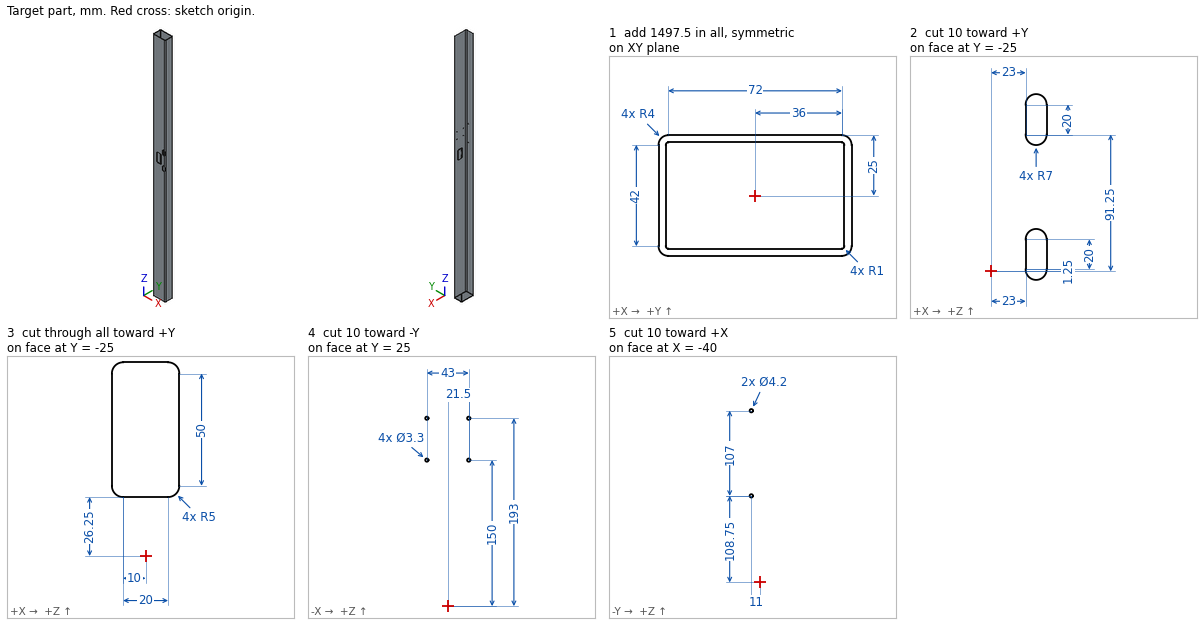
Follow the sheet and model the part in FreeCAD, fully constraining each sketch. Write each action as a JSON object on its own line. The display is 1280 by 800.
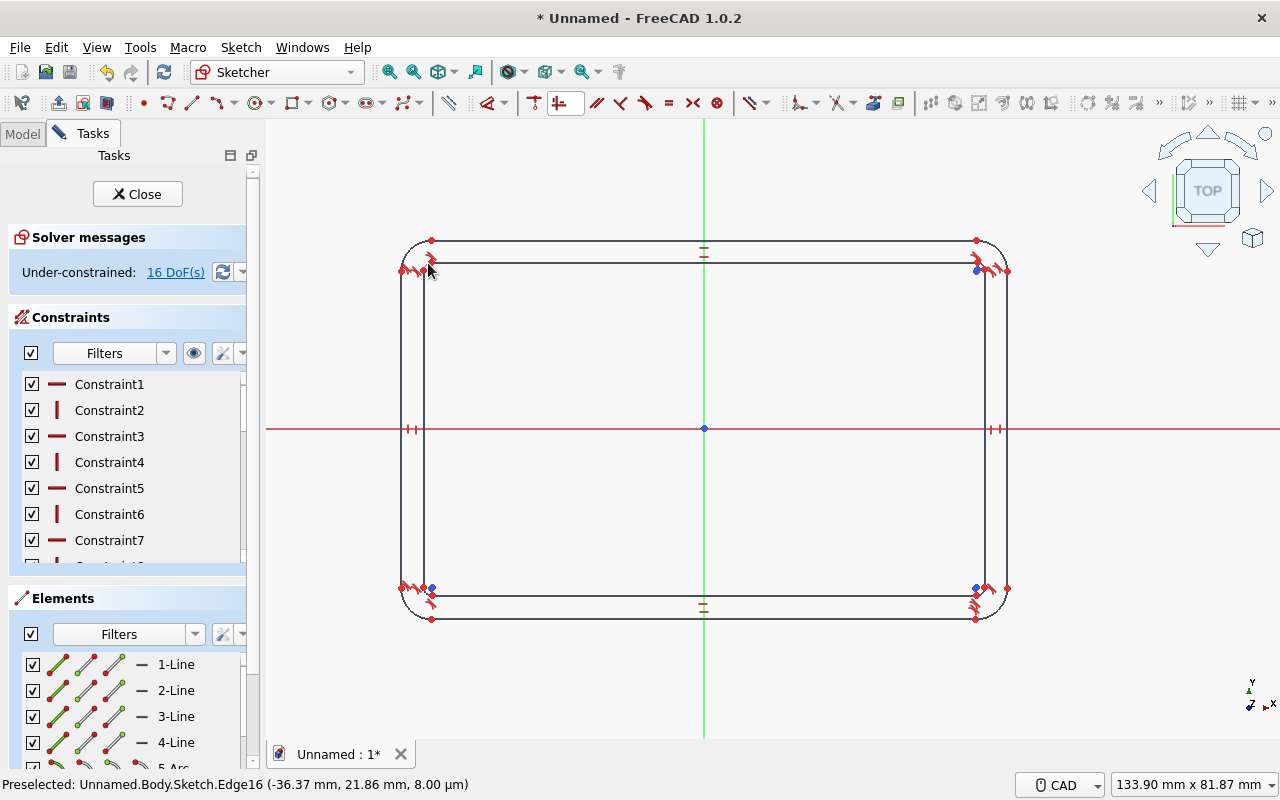
{"action": "left_click", "coordinate": [1004, 257]}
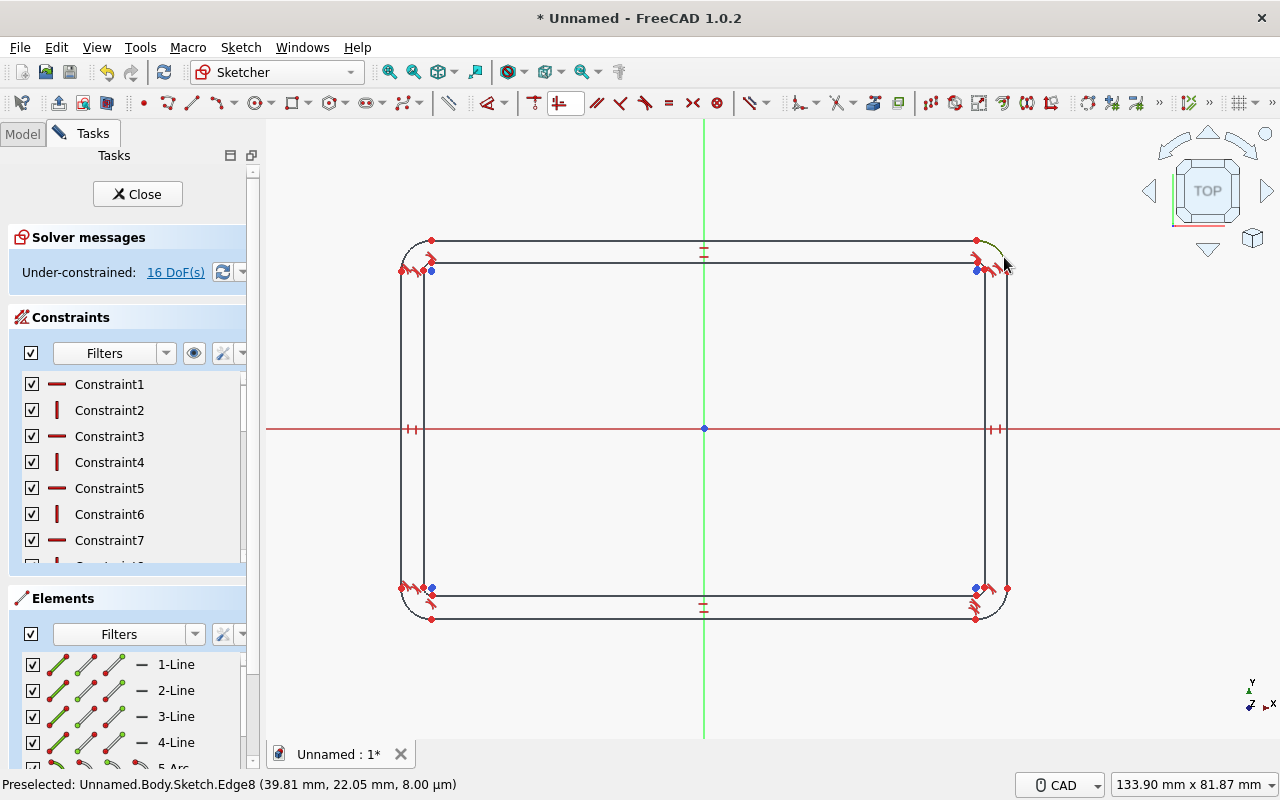
{"action": "scroll", "coordinate": [983, 265], "scroll_direction": "up", "scroll_amount": 5}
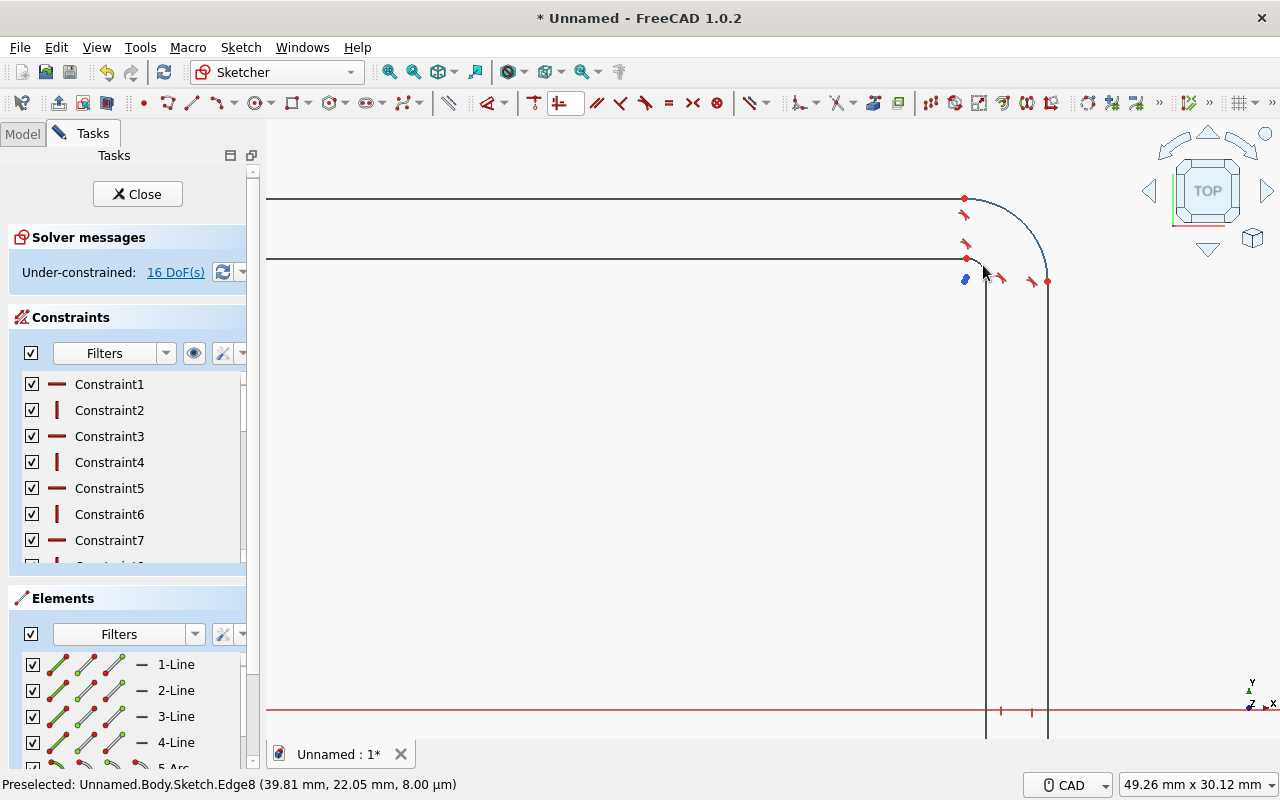
{"action": "left_click", "coordinate": [981, 264]}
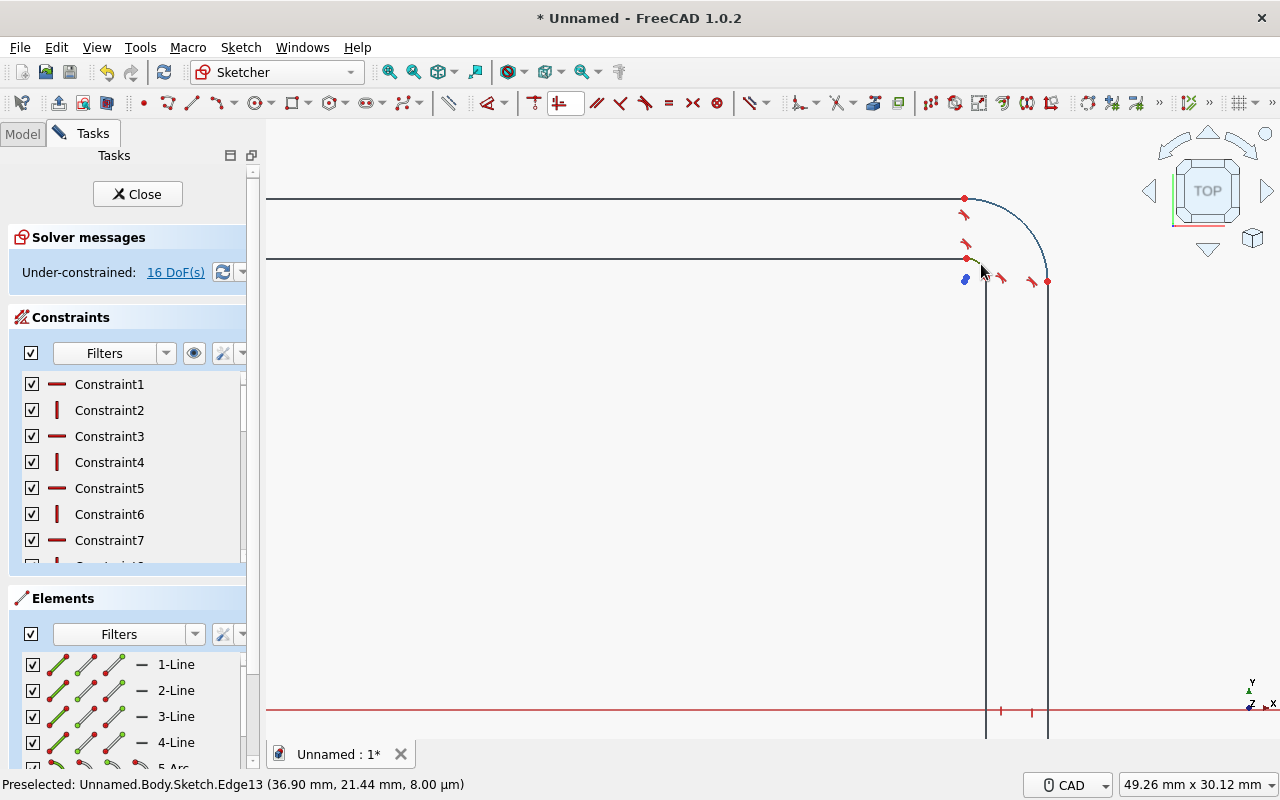
{"action": "key", "text": "c"}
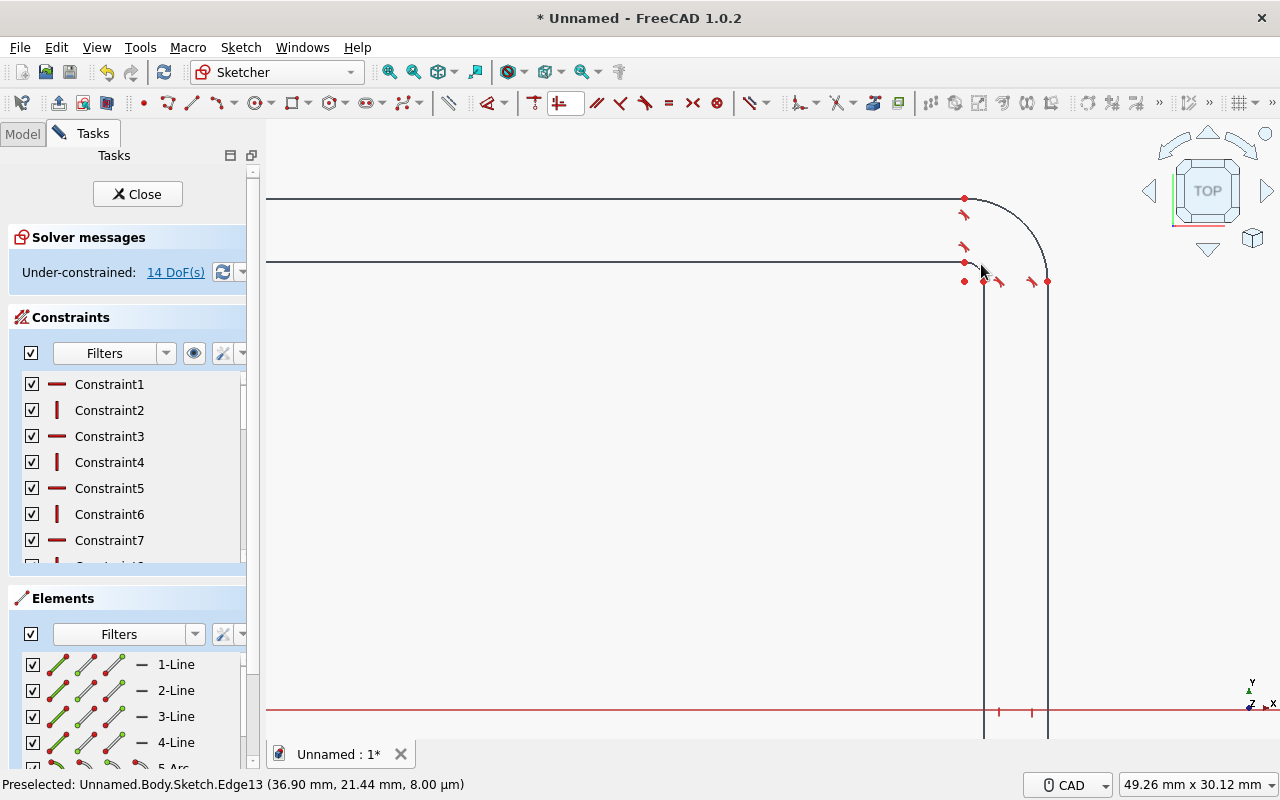
{"action": "scroll", "coordinate": [984, 265], "scroll_direction": "down", "scroll_amount": 5}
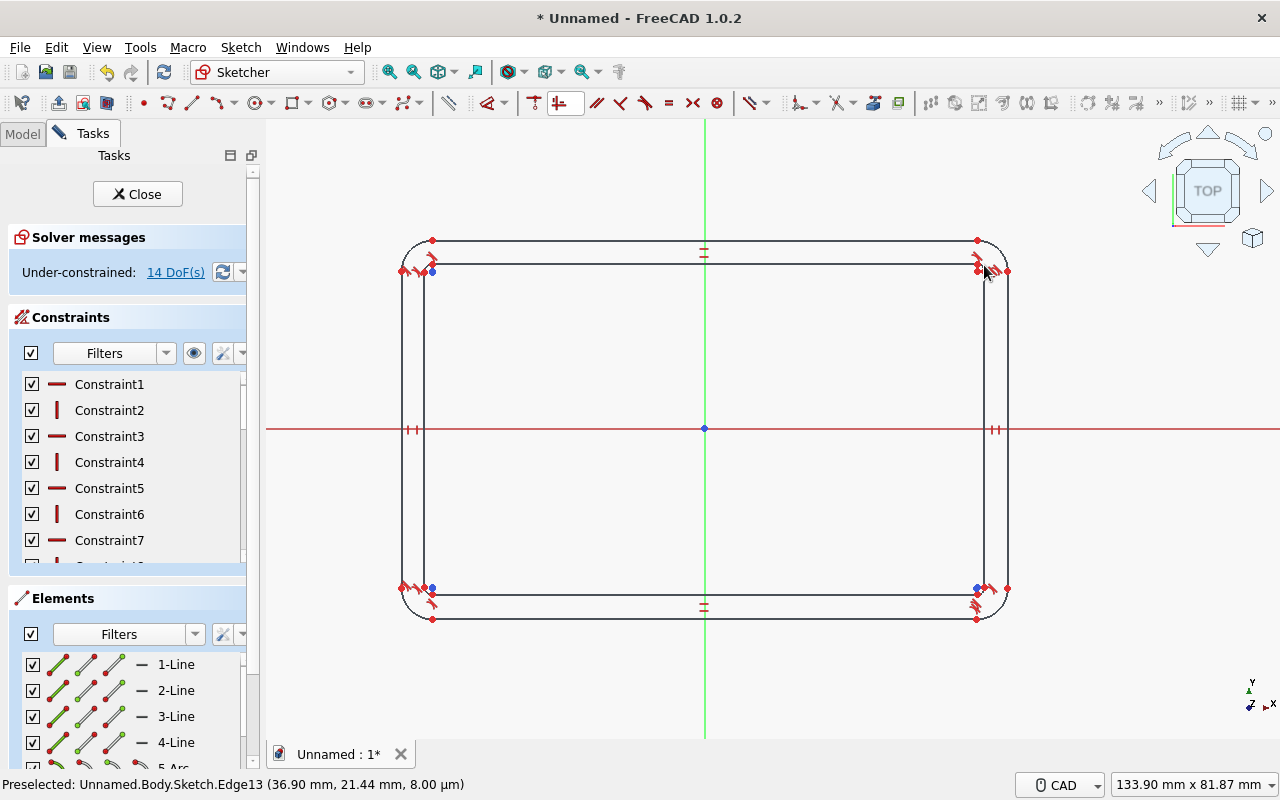
{"action": "left_click", "coordinate": [991, 616]}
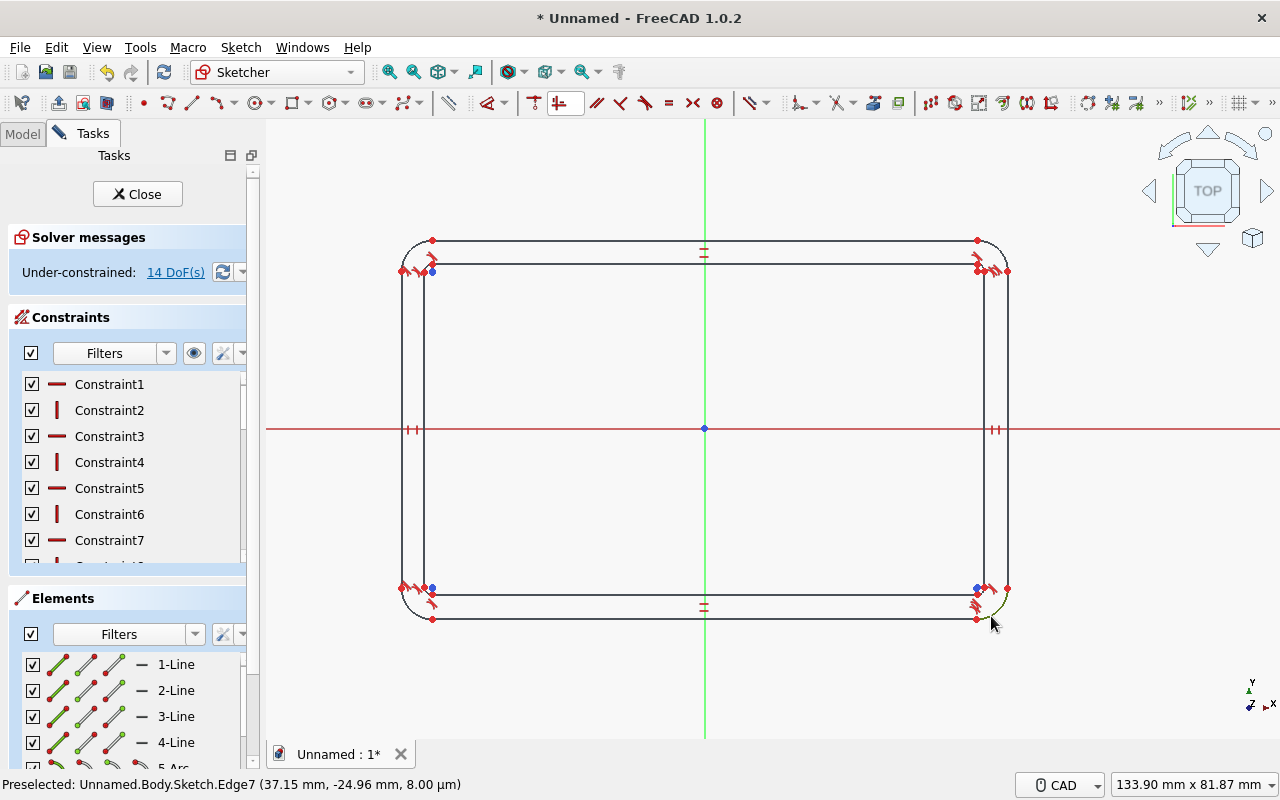
{"action": "scroll", "coordinate": [982, 593], "scroll_direction": "up", "scroll_amount": 5}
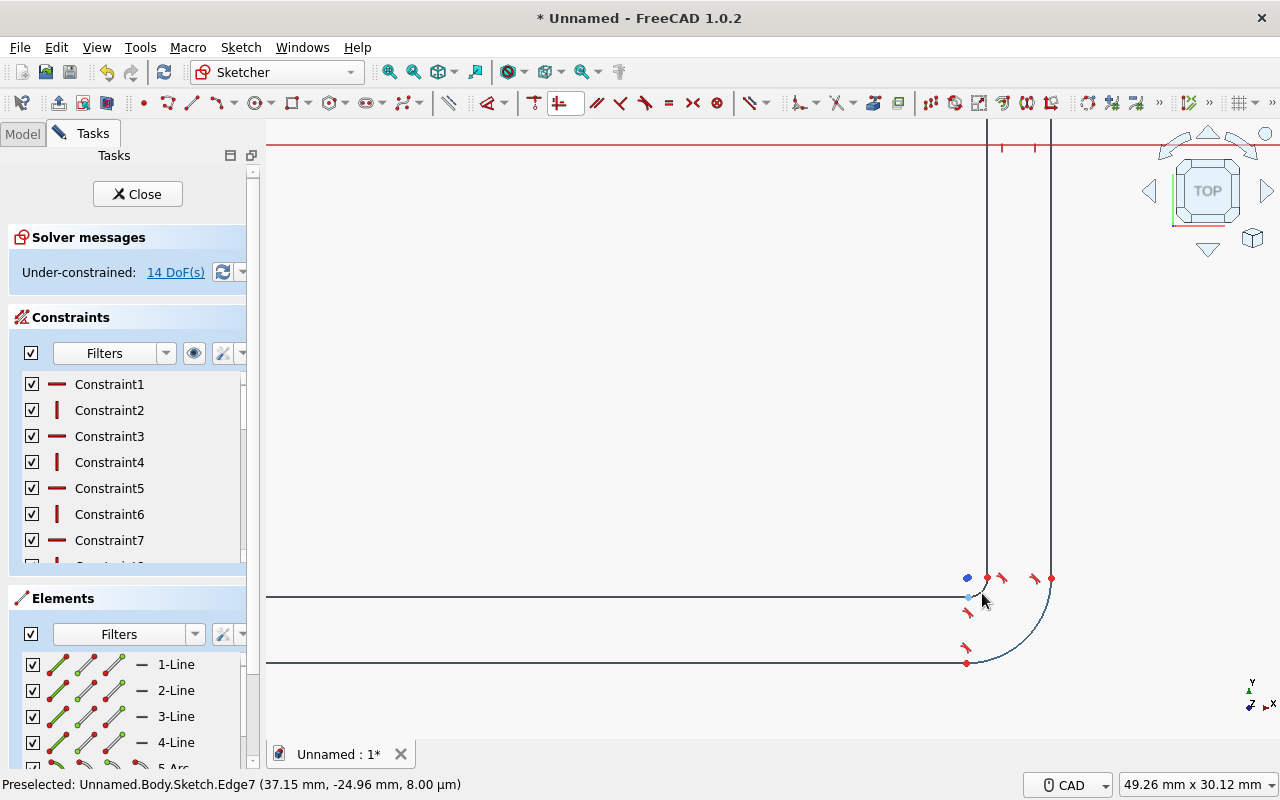
{"action": "left_click", "coordinate": [982, 591]}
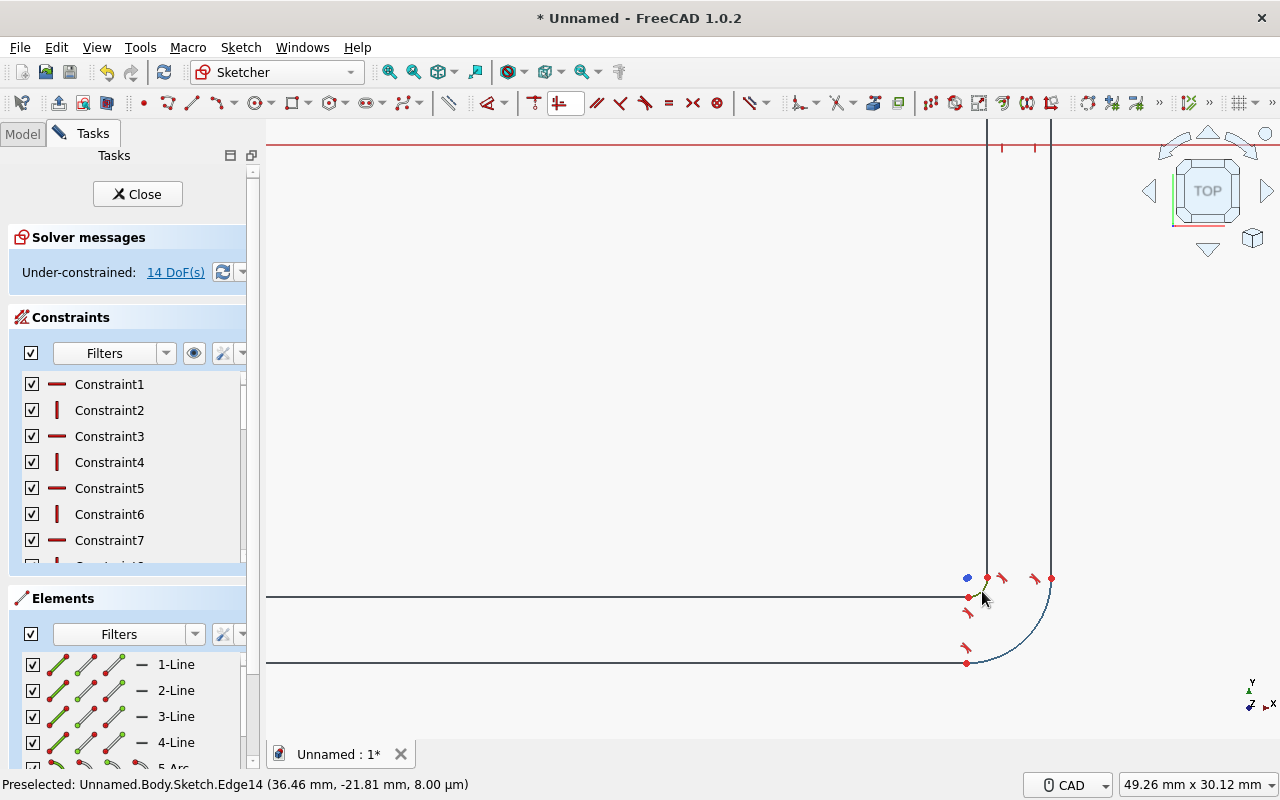
{"action": "key", "text": "c"}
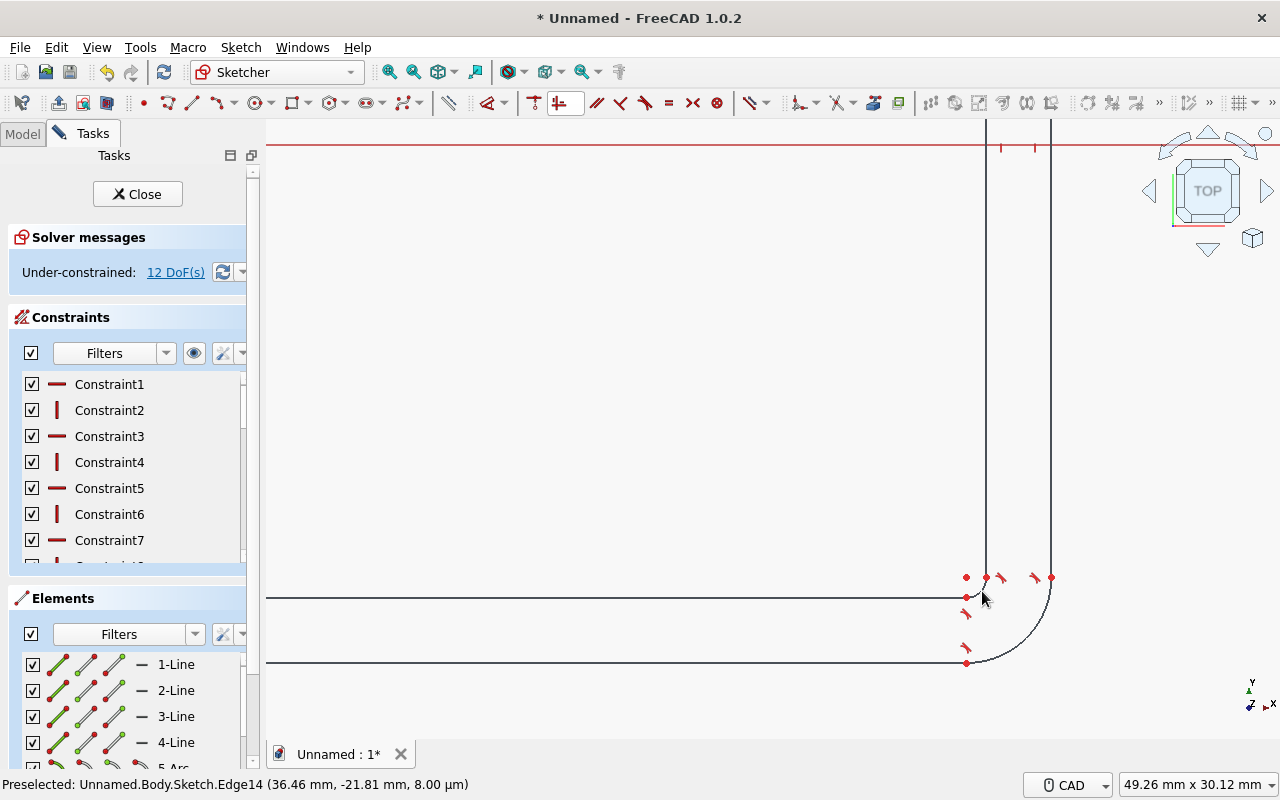
{"action": "scroll", "coordinate": [982, 594], "scroll_direction": "down", "scroll_amount": 5}